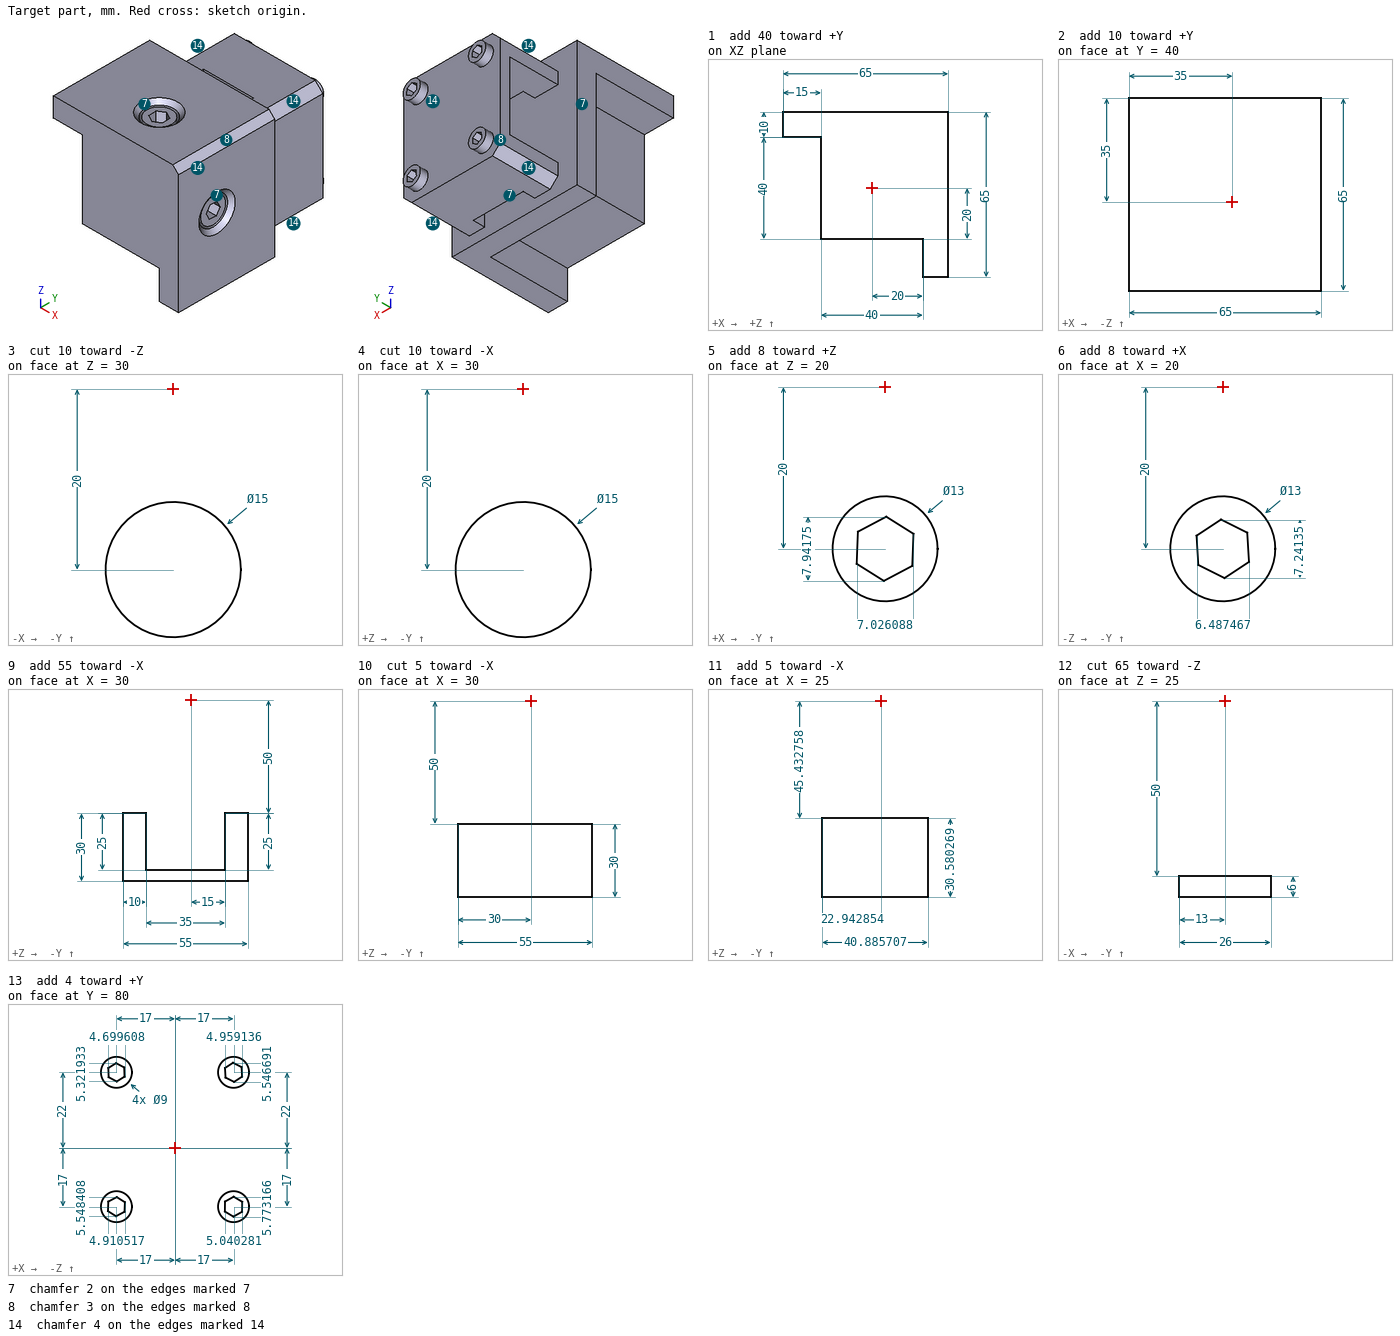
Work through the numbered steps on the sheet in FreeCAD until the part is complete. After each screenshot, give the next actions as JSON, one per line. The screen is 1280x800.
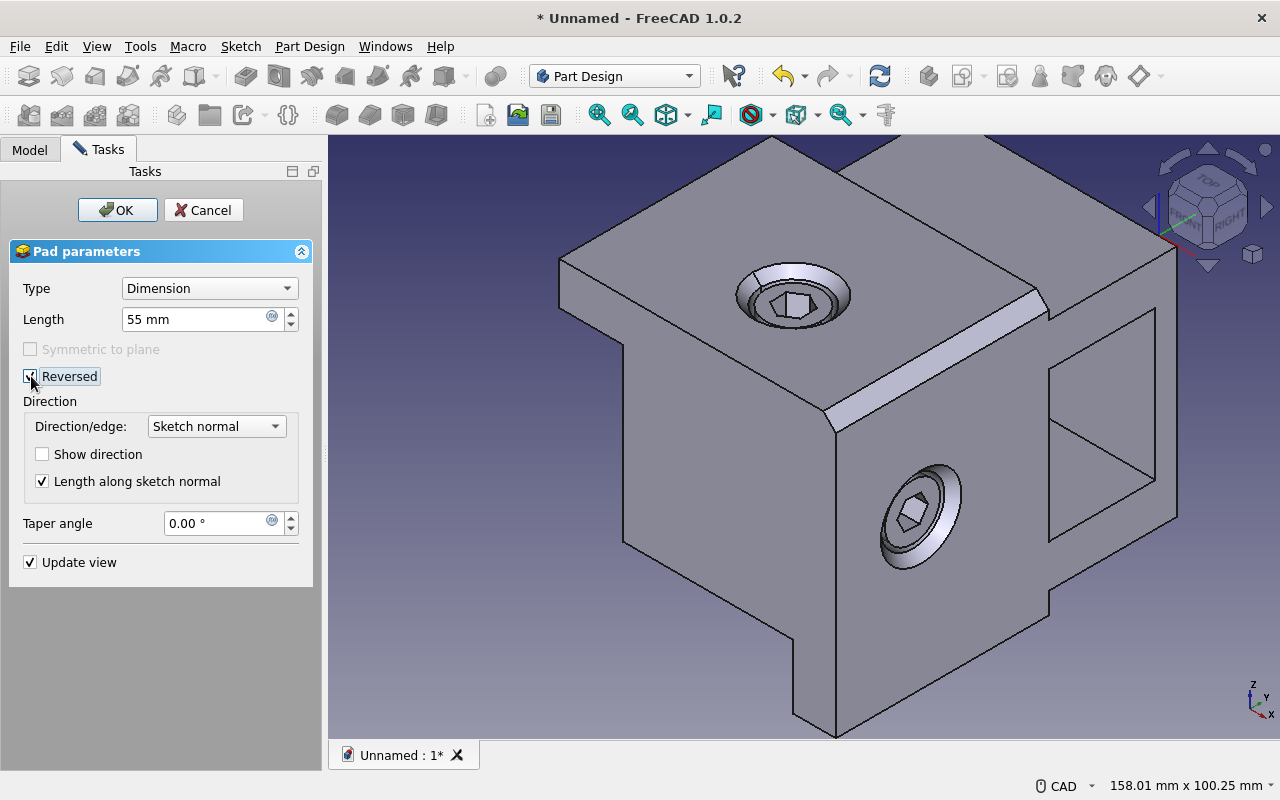
{"action": "left_click", "coordinate": [118, 210]}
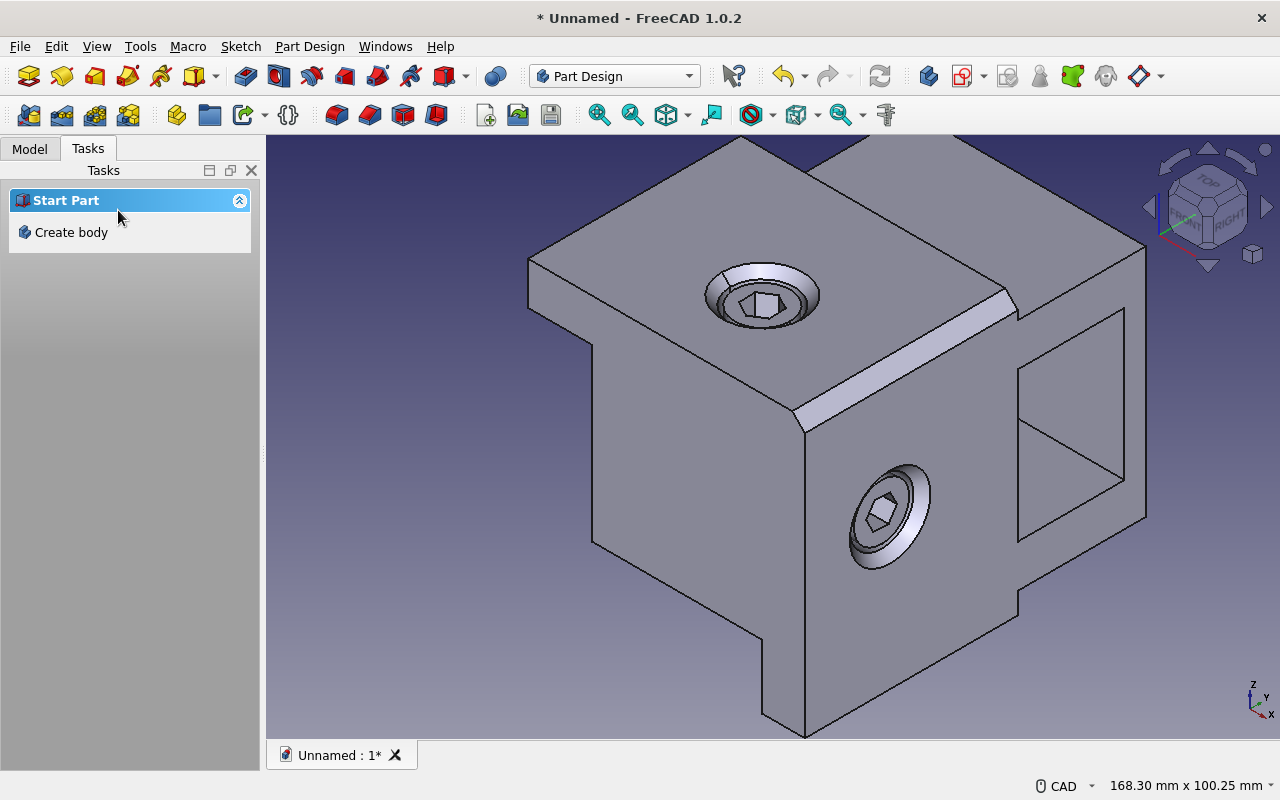
{"action": "left_click", "coordinate": [600, 116]}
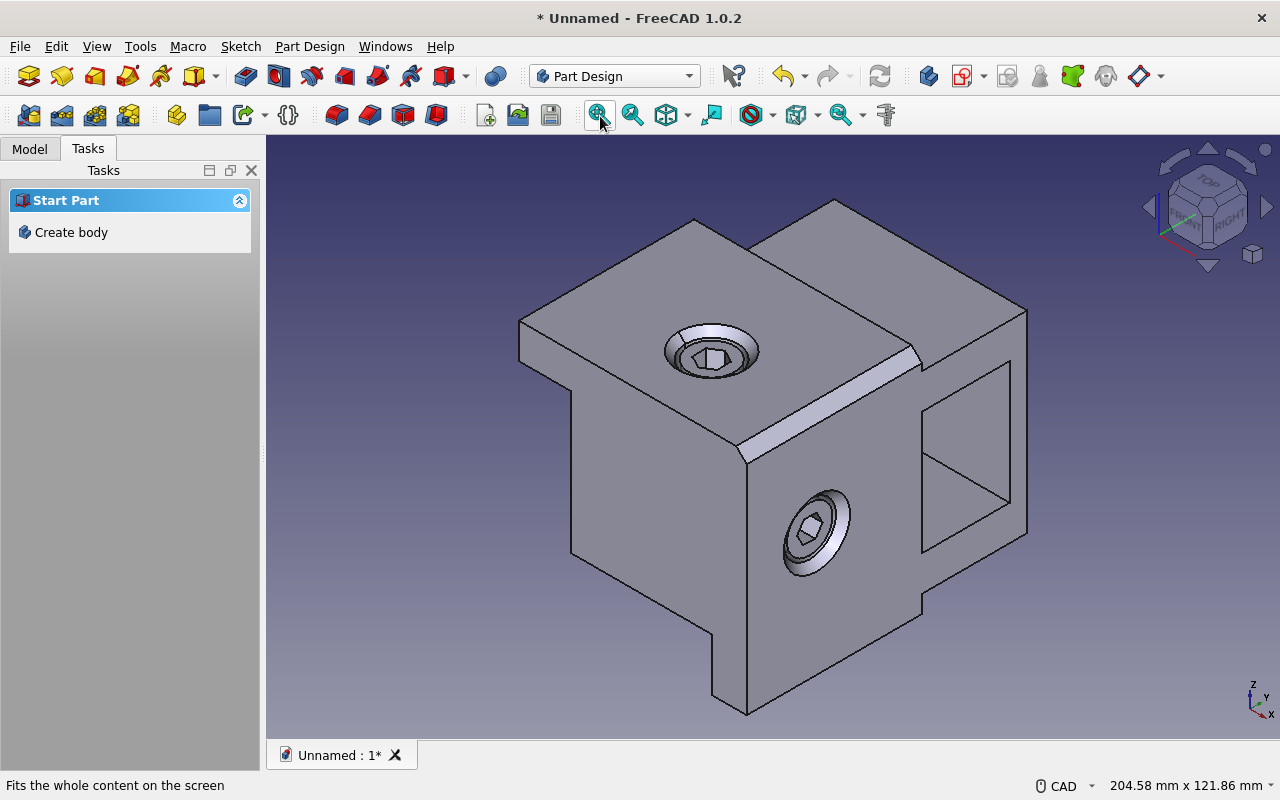
{"action": "left_click", "coordinate": [847, 603]}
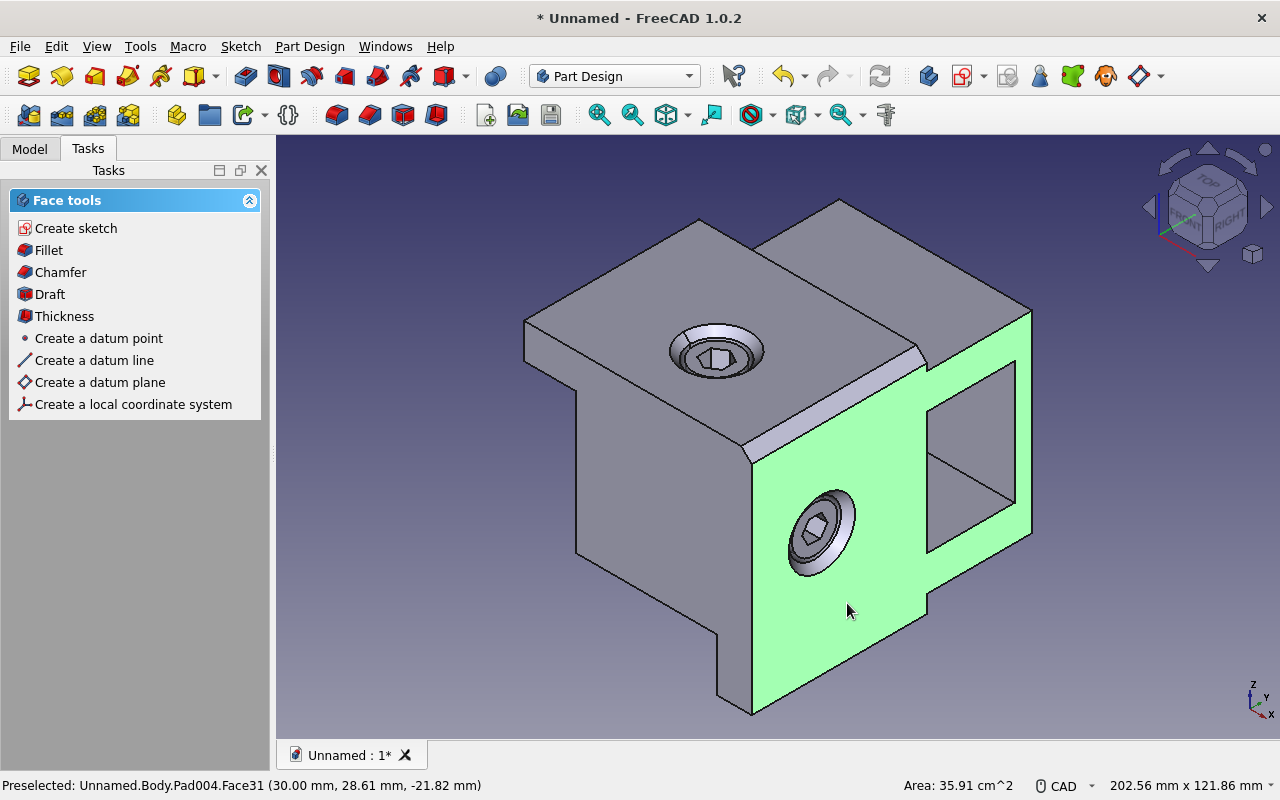
{"action": "left_click", "coordinate": [962, 76]}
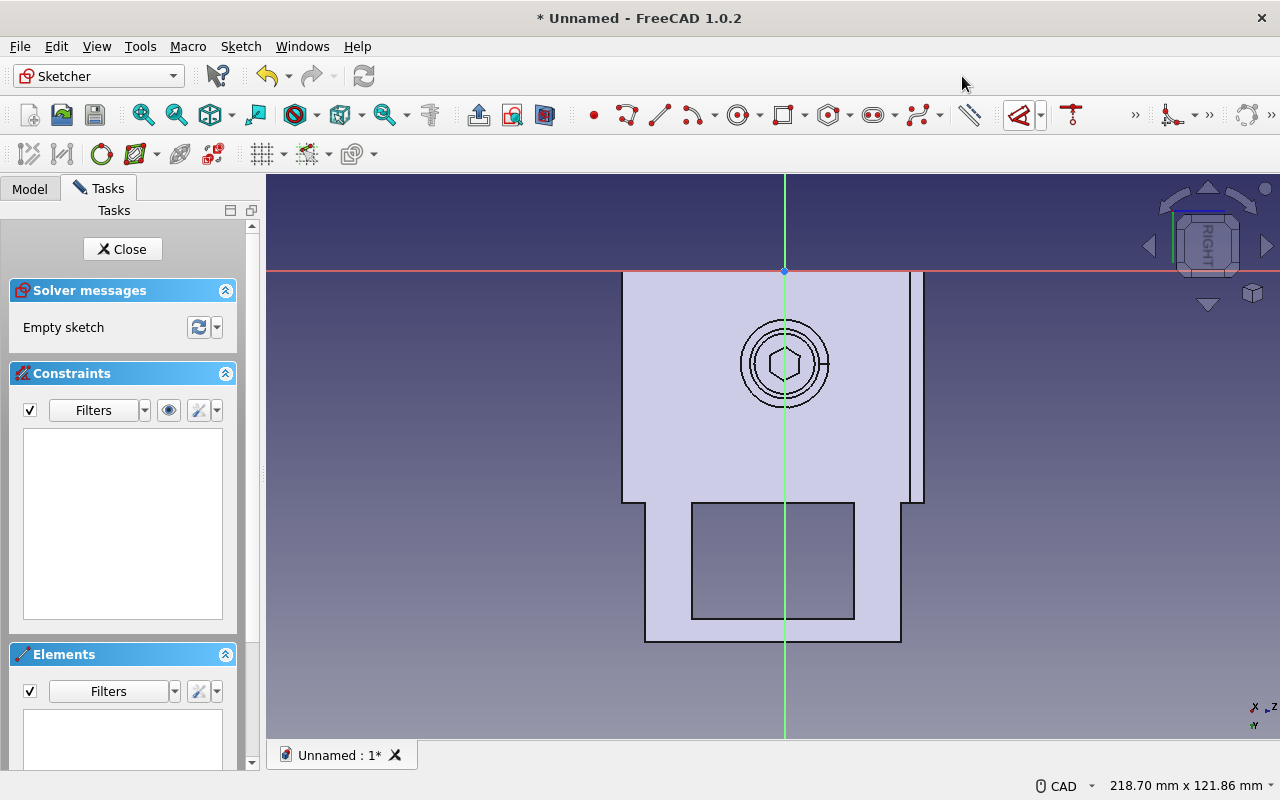
{"action": "left_click", "coordinate": [782, 116]}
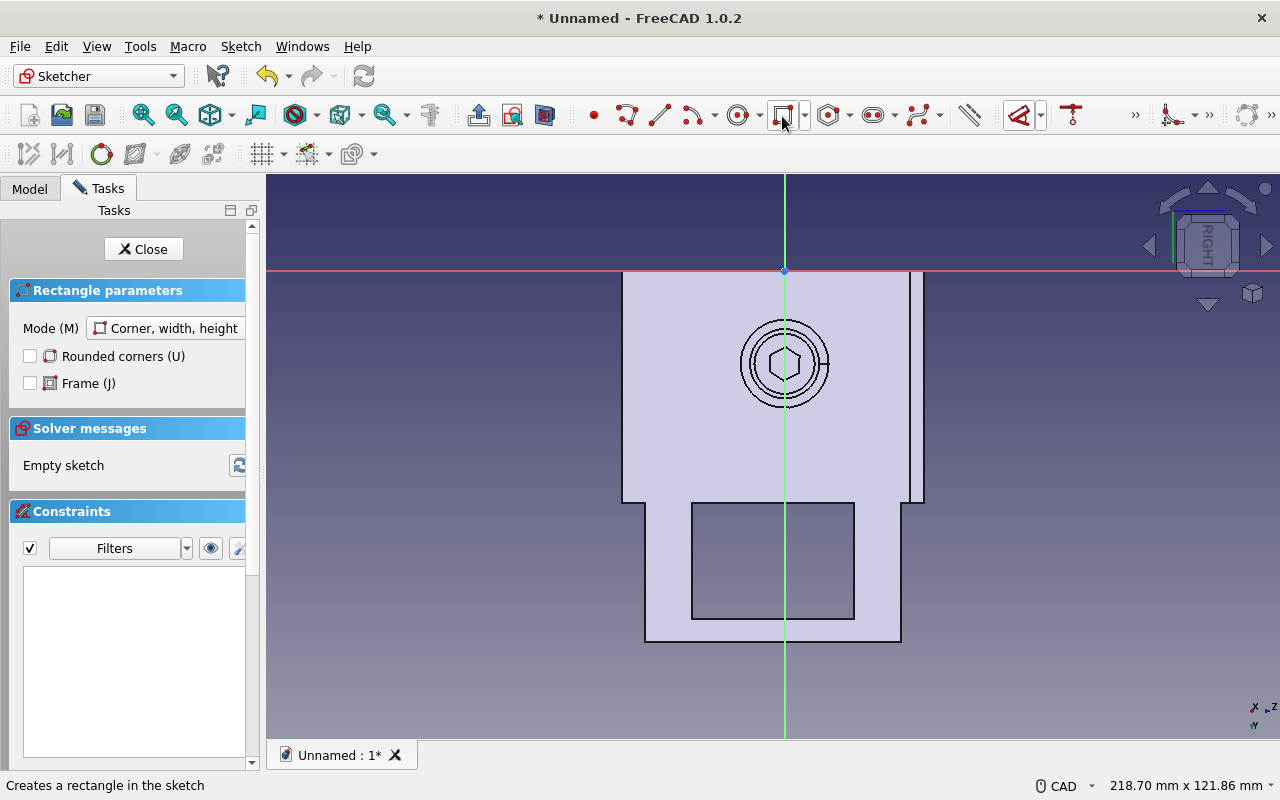
{"action": "left_click", "coordinate": [645, 503]}
{"action": "mouse_move", "coordinate": [901, 642]}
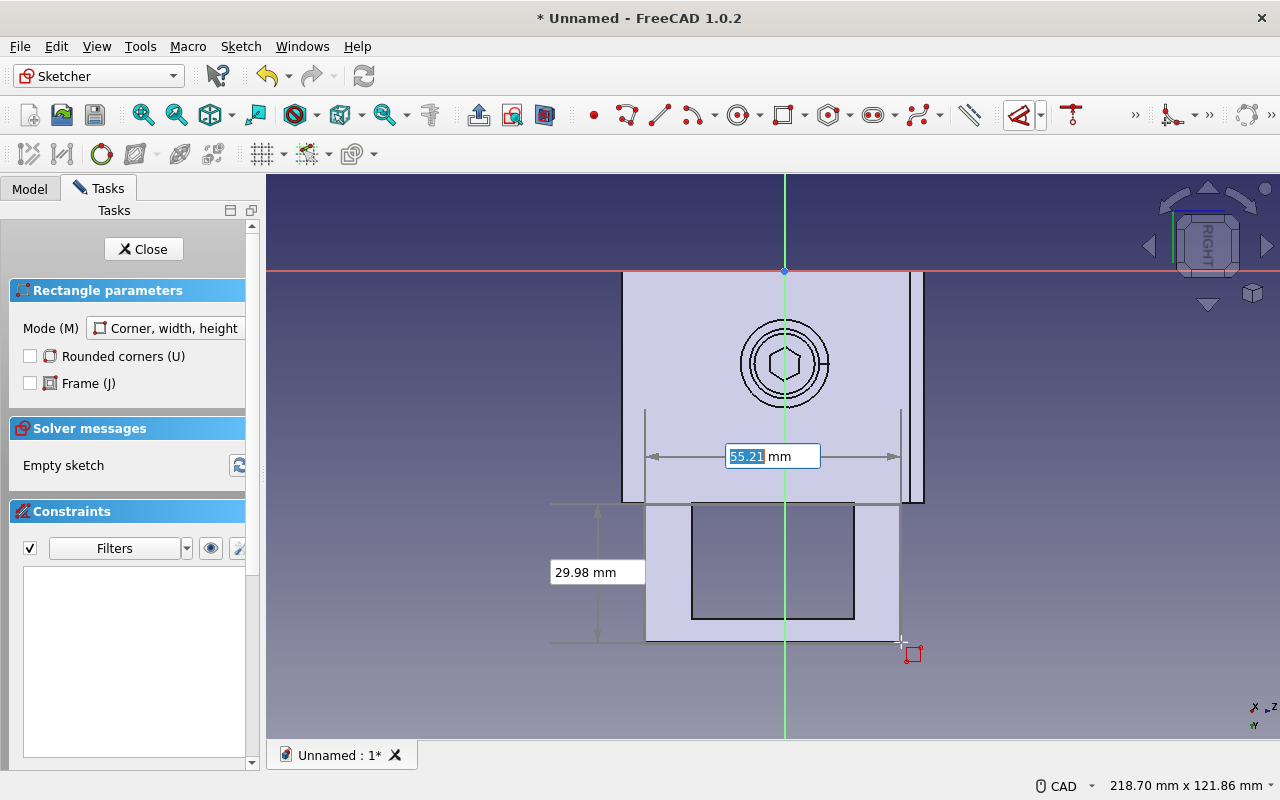
{"action": "type", "text": "55"}
{"action": "key", "text": "Tab"}
{"action": "type", "text": "30"}
{"action": "key", "text": "Return"}
{"action": "key", "text": "Escape"}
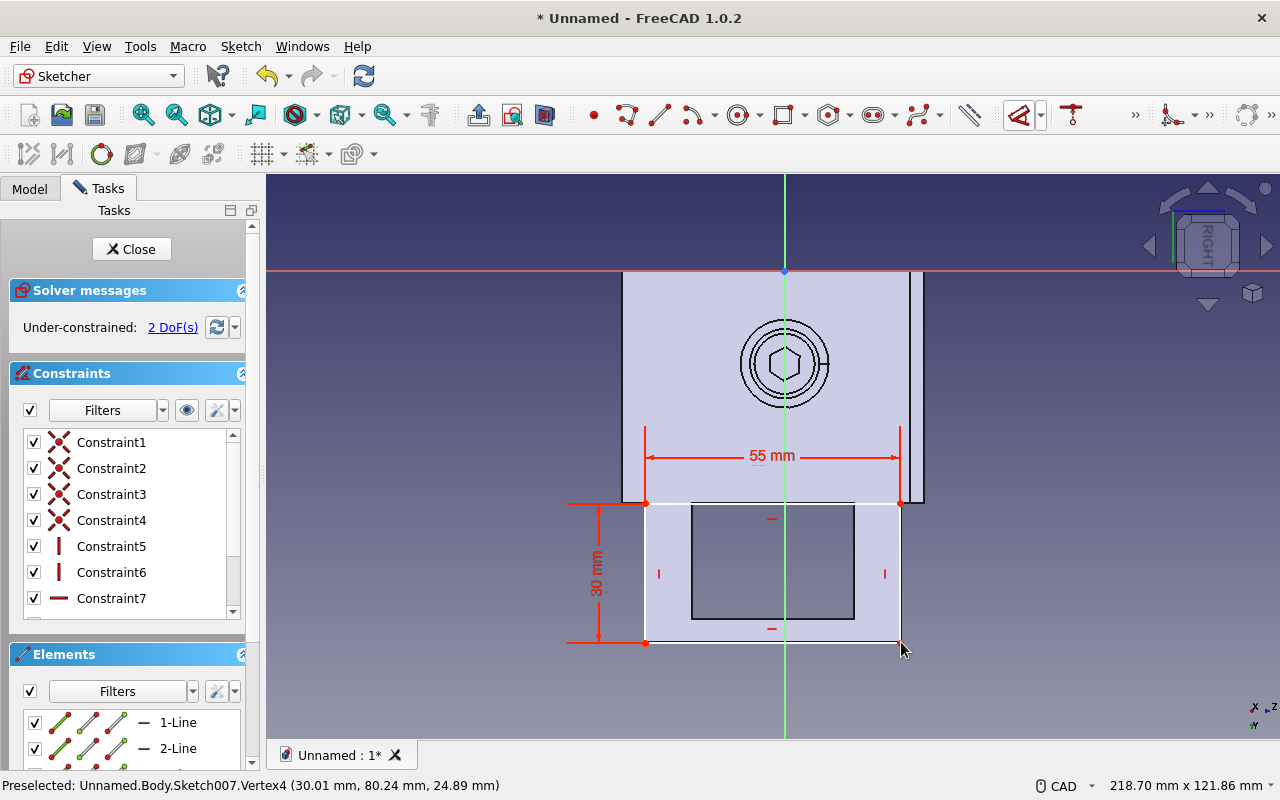
{"action": "left_click", "coordinate": [645, 504]}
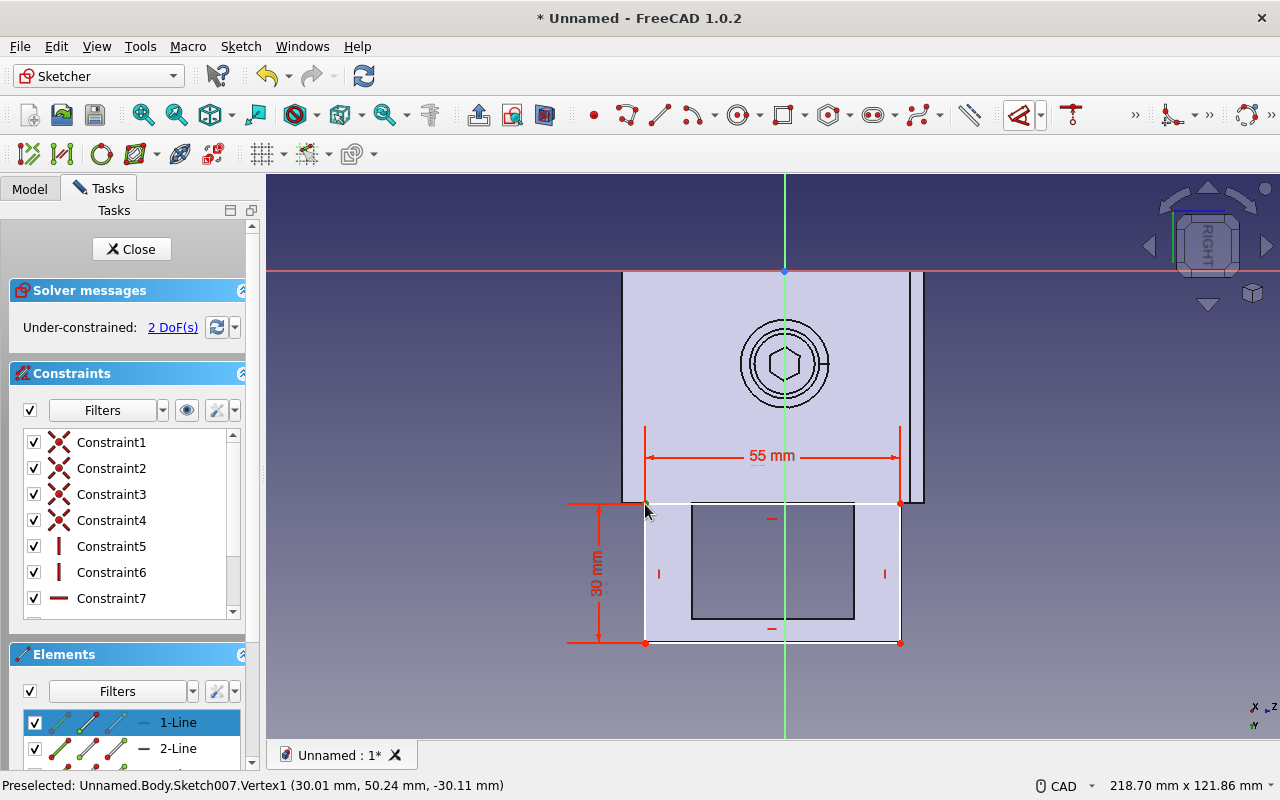
{"action": "left_click", "coordinate": [1040, 116]}